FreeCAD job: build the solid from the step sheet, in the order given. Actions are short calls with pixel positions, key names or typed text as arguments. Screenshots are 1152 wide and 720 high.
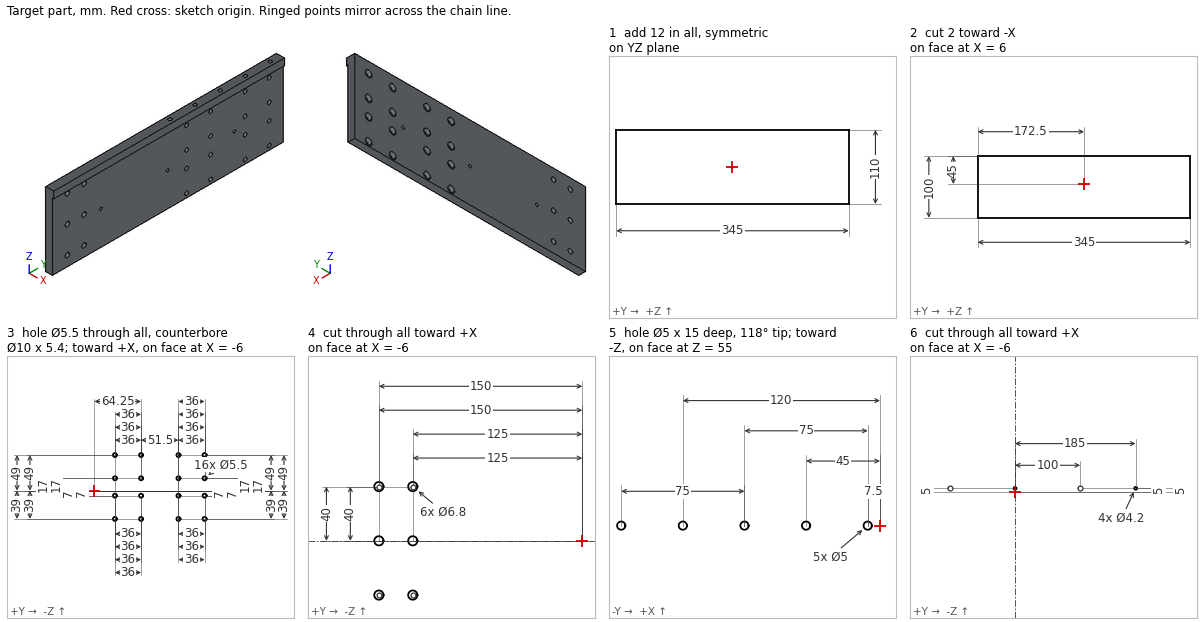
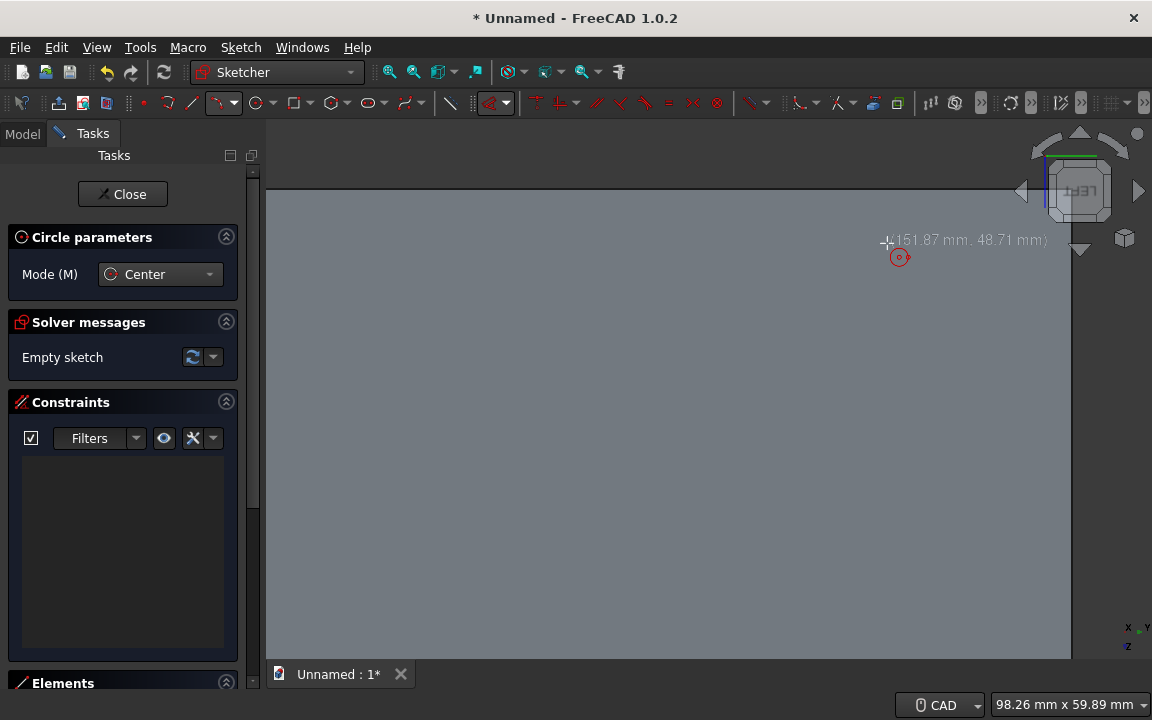
click(885, 243)
click(902, 225)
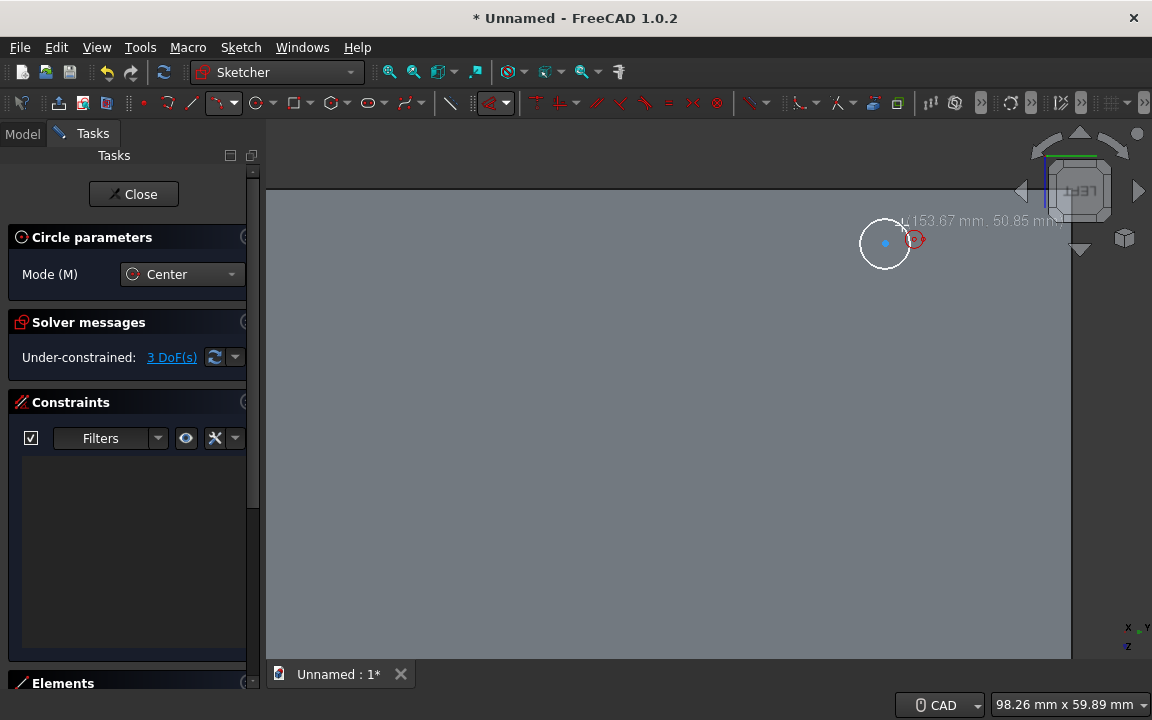
click(885, 531)
click(902, 514)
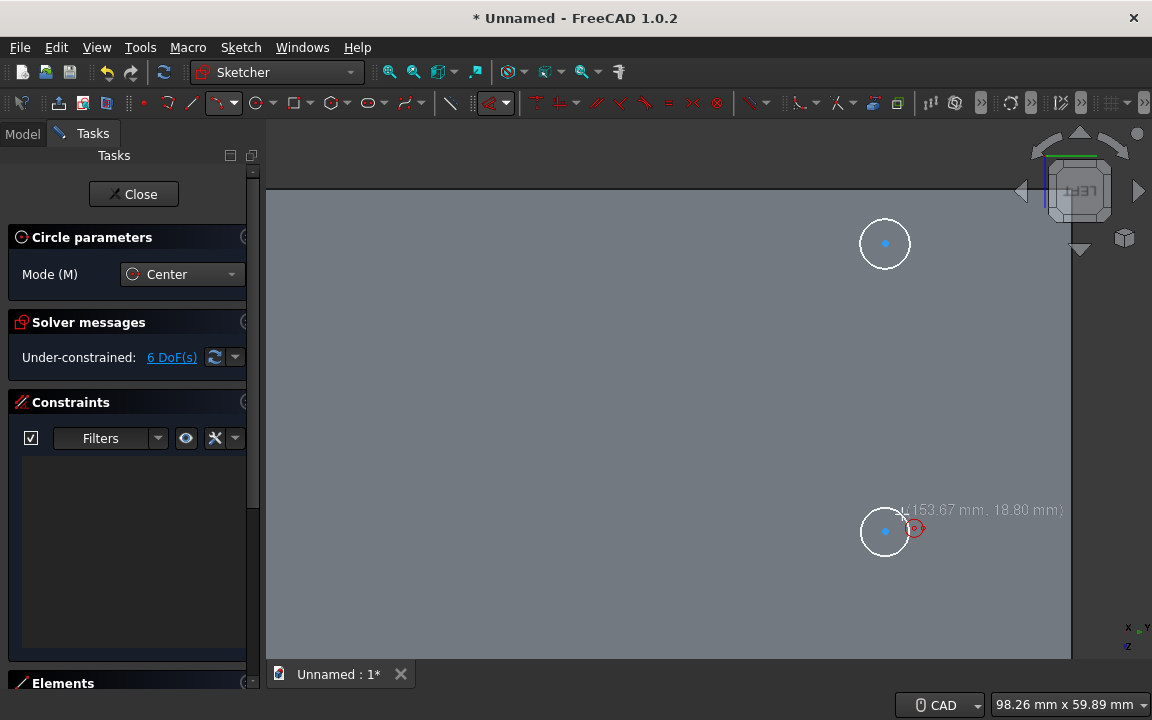
scroll(889, 243, down, 5)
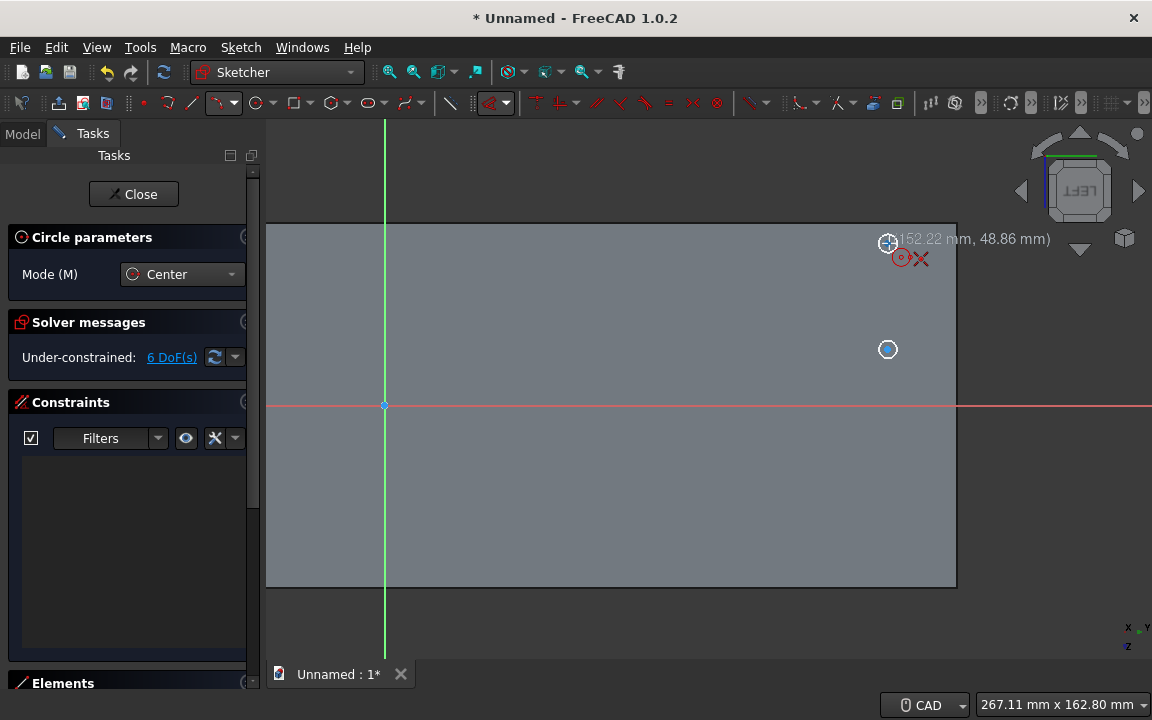
scroll(888, 429, up, 5)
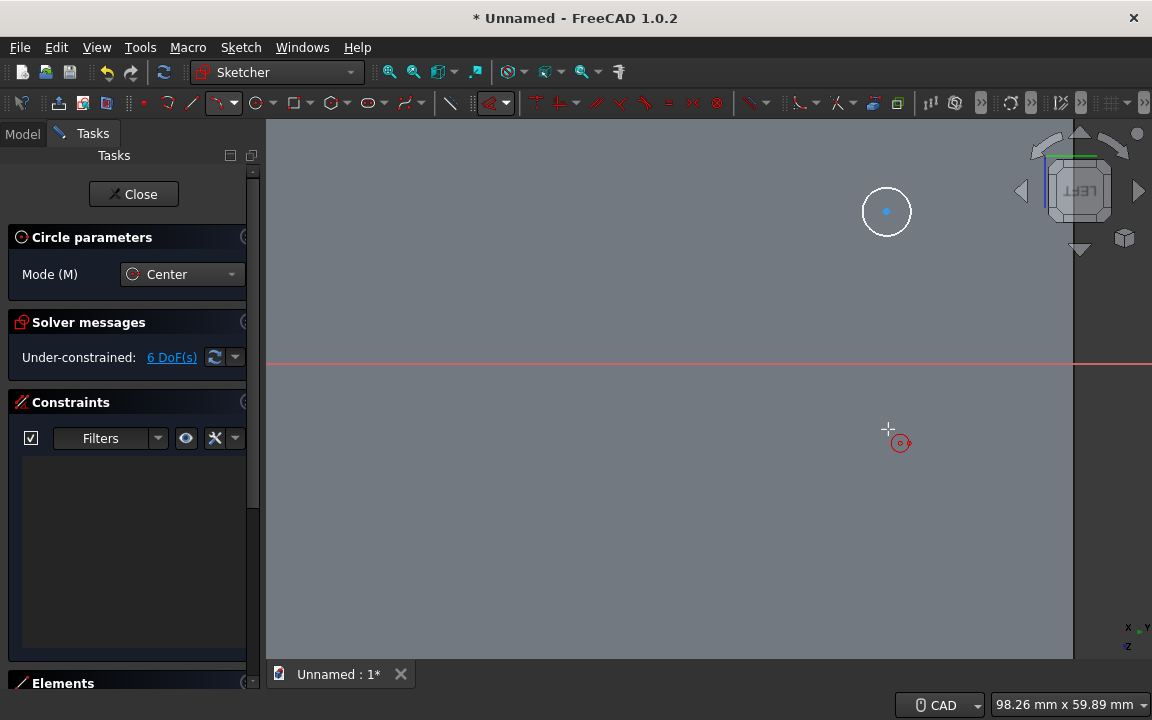
click(886, 427)
click(904, 410)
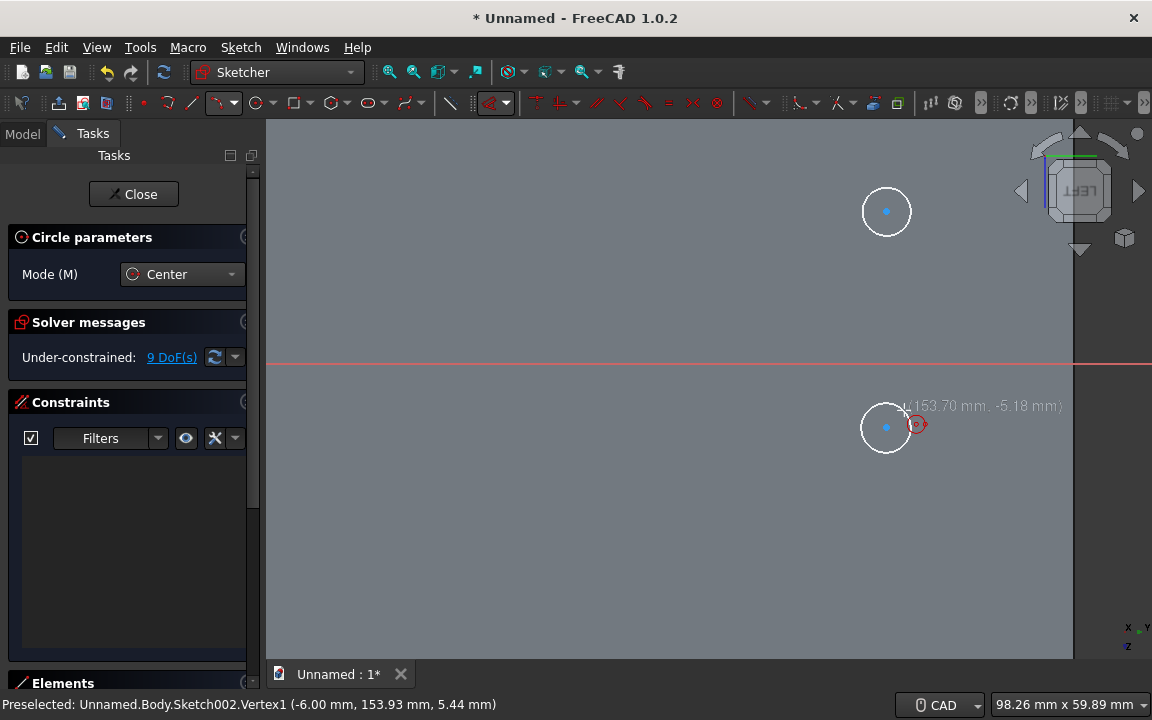
scroll(888, 430, down, 5)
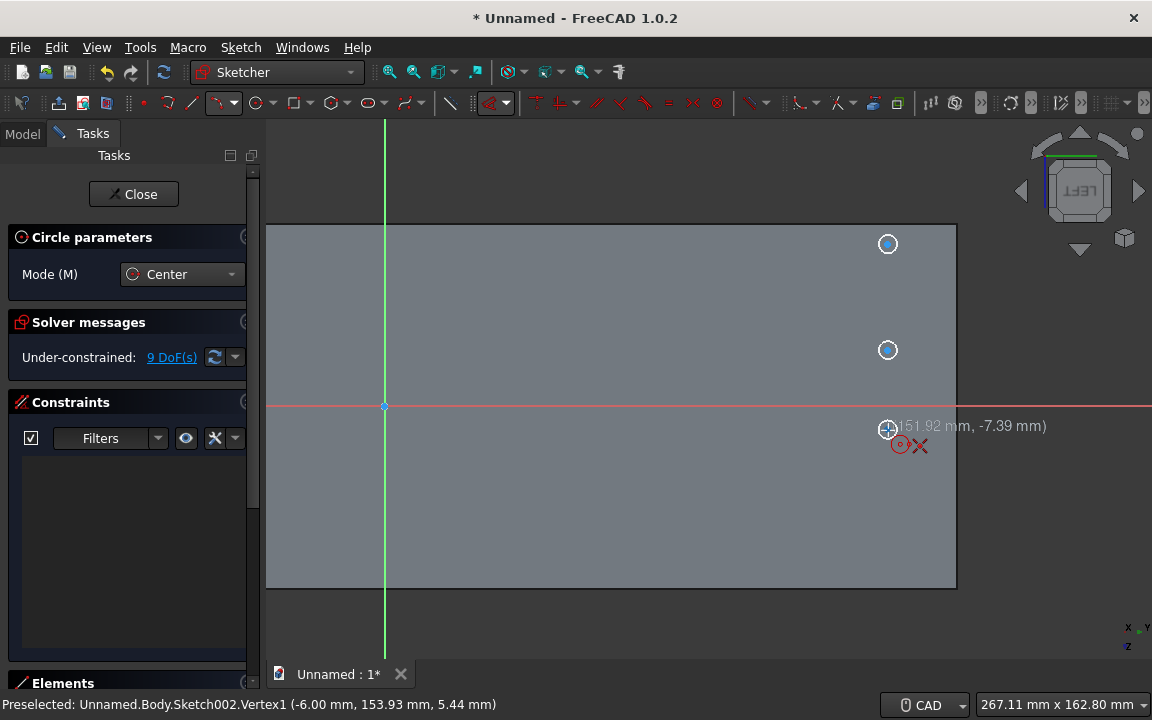
scroll(888, 536, up, 5)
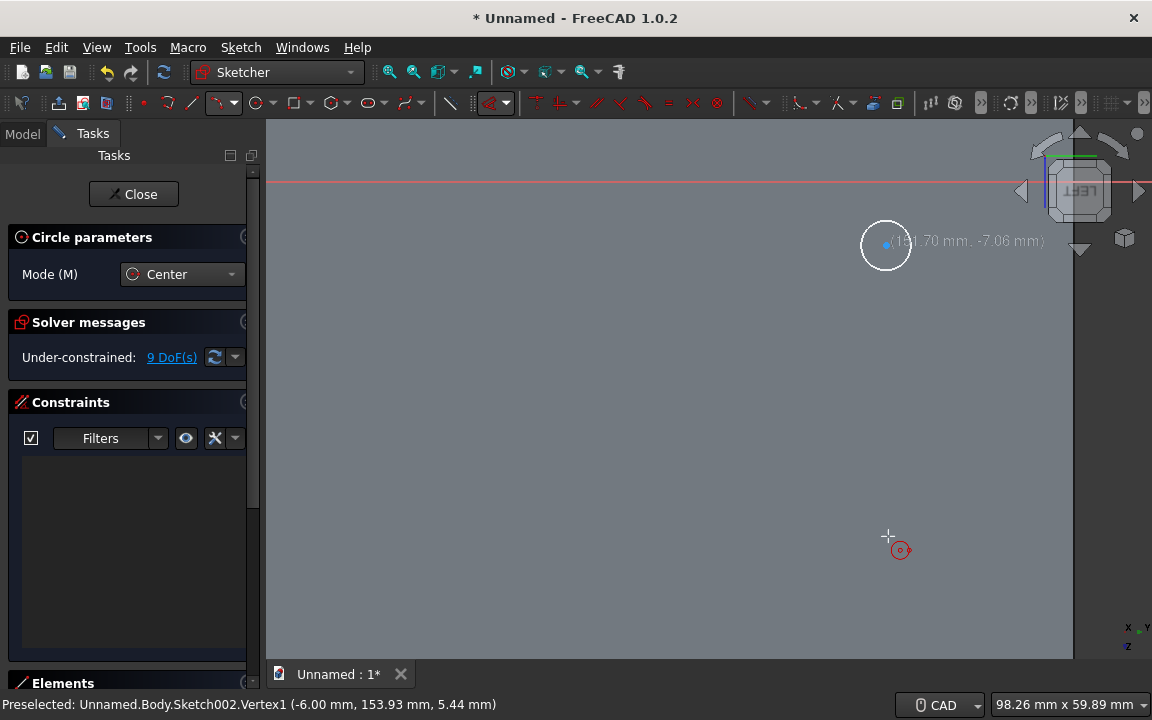
click(886, 534)
click(904, 516)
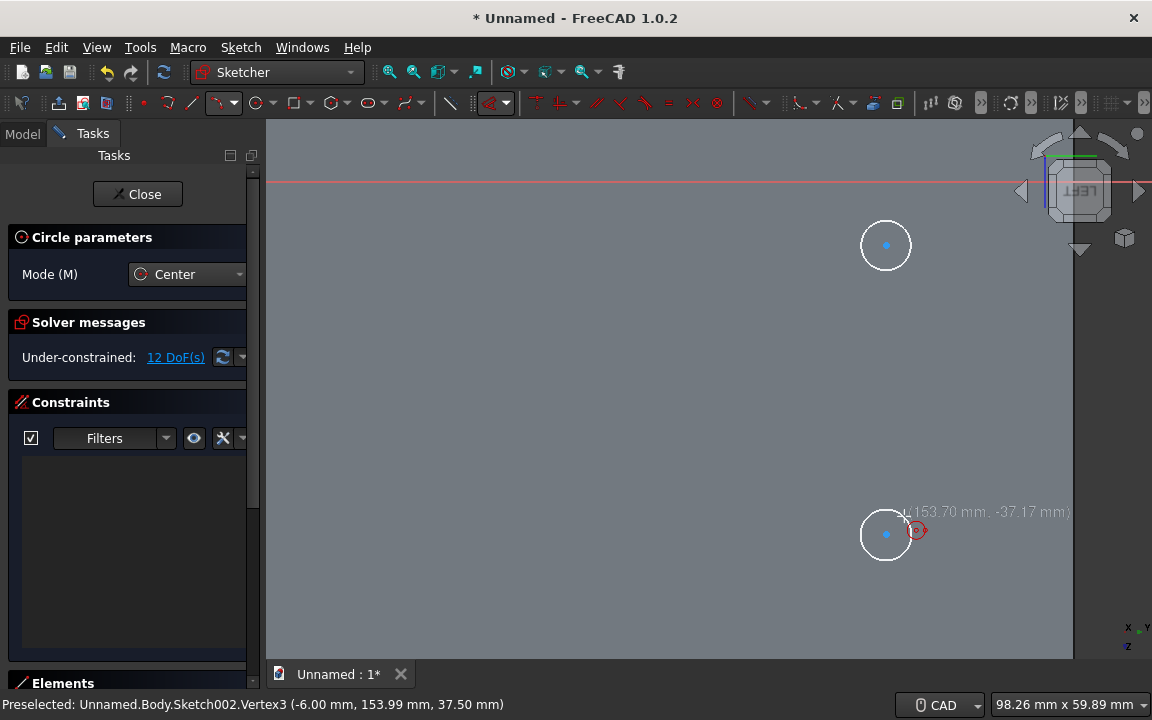
click(562, 534)
click(579, 516)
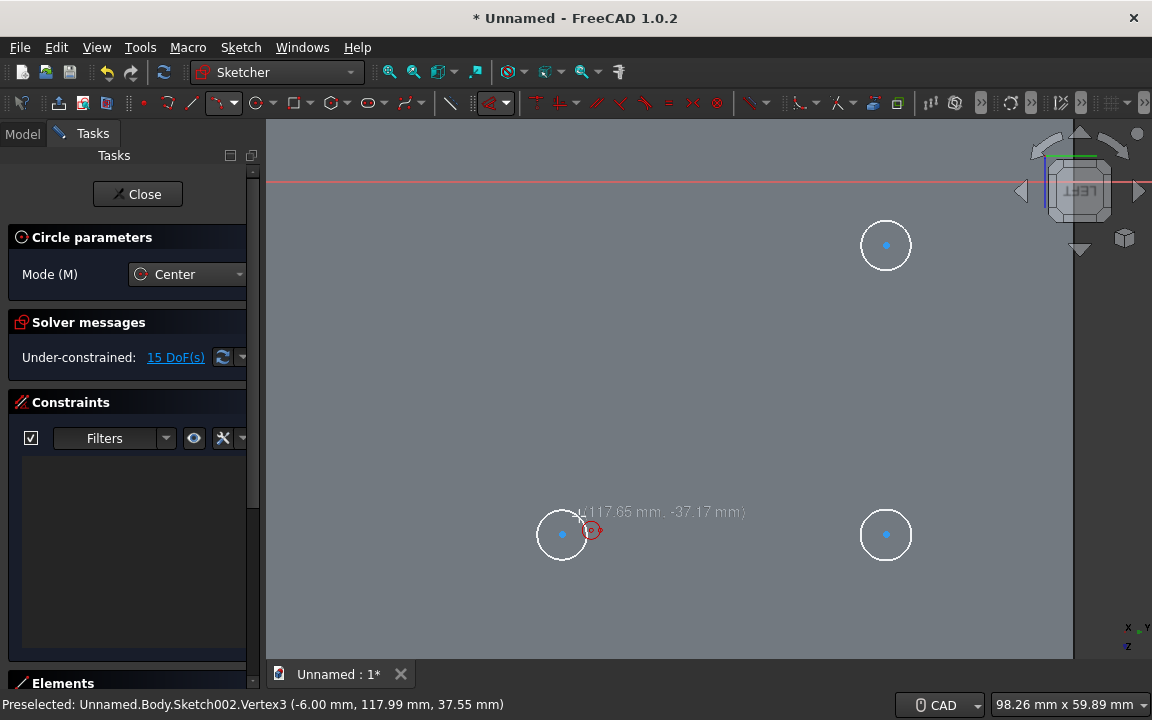
click(562, 245)
click(579, 227)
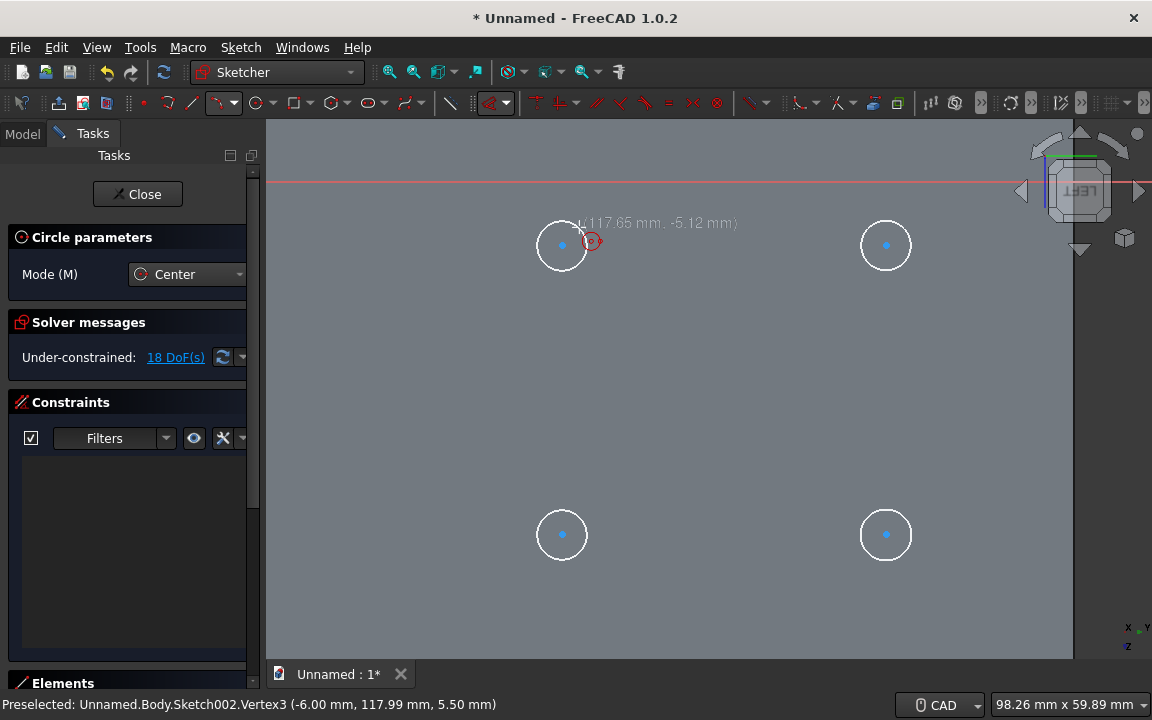
scroll(888, 536, down, 5)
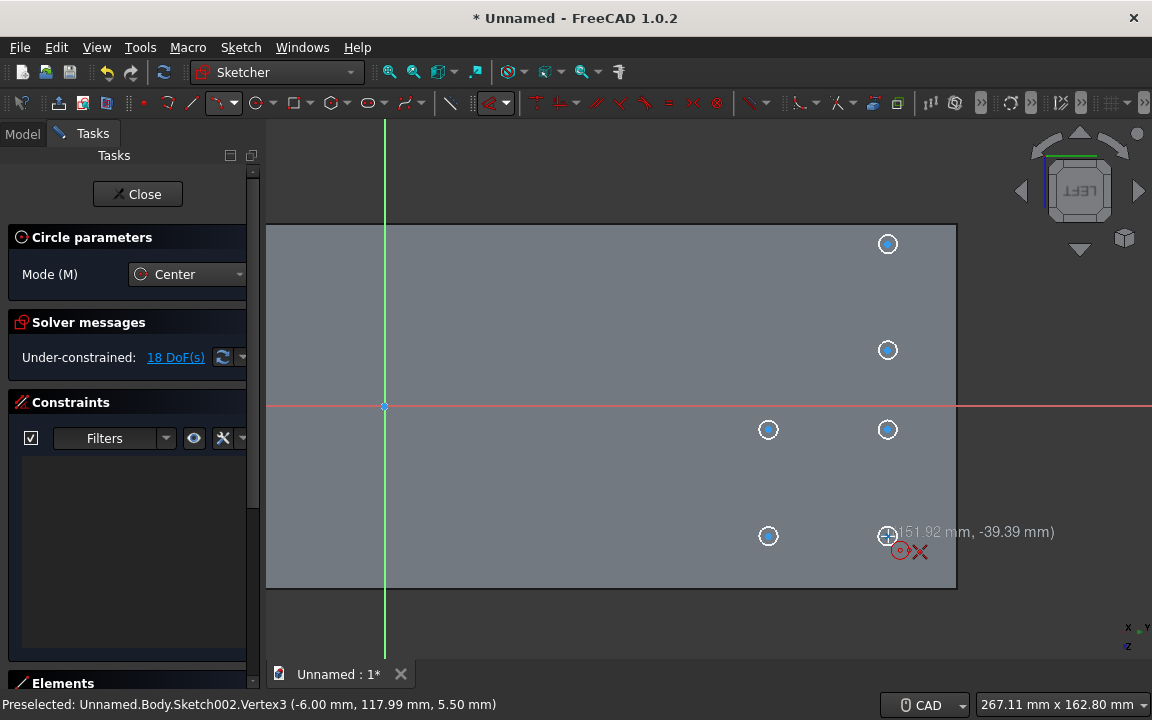
scroll(768, 350, up, 5)